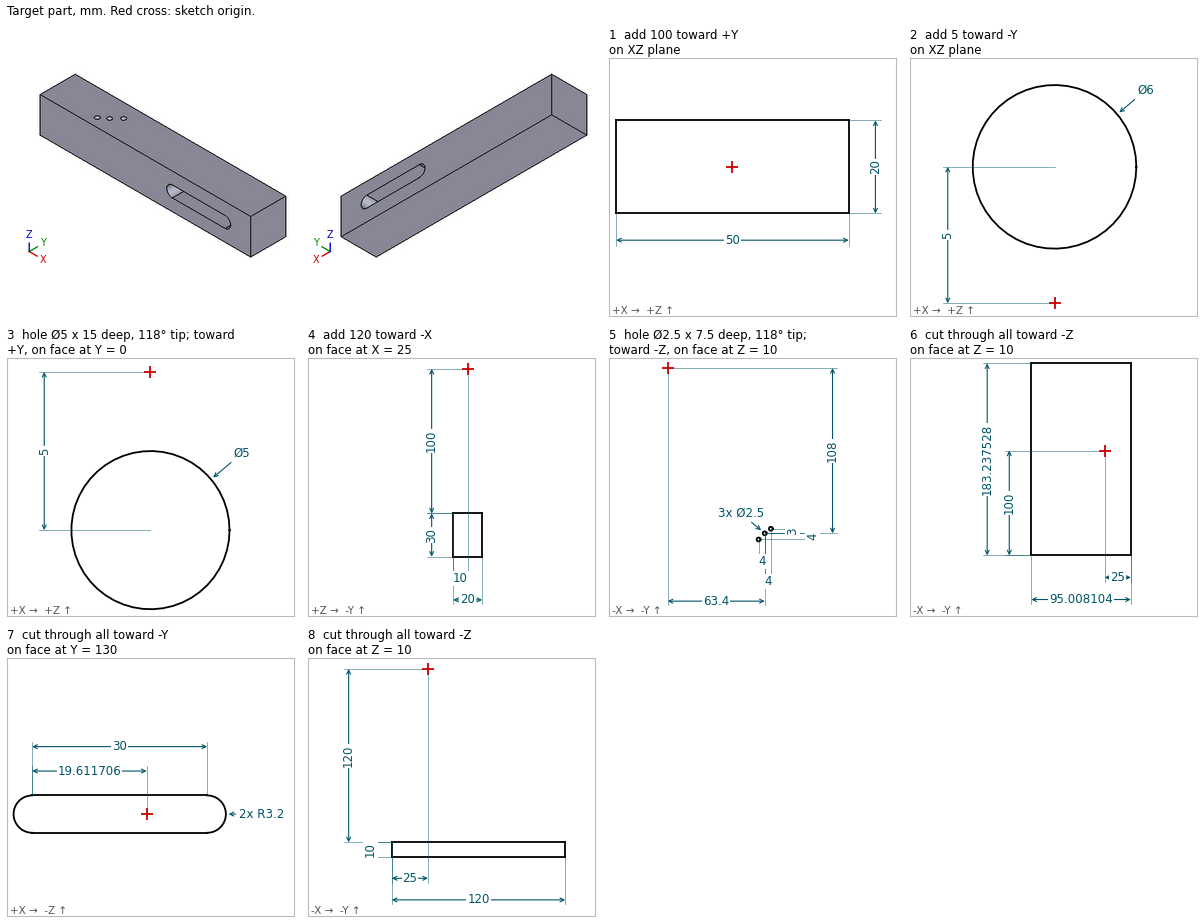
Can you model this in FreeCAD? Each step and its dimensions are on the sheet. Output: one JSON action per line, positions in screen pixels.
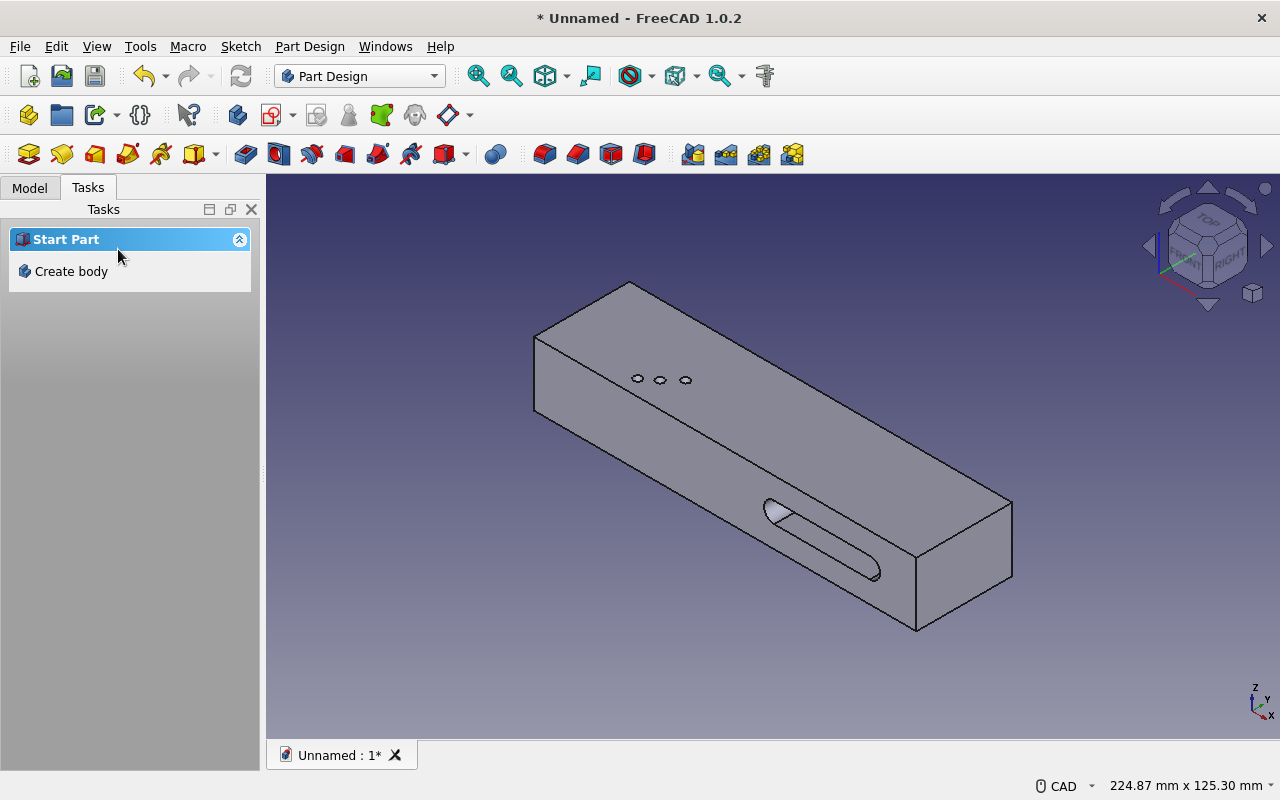
{"action": "left_click", "coordinate": [882, 482]}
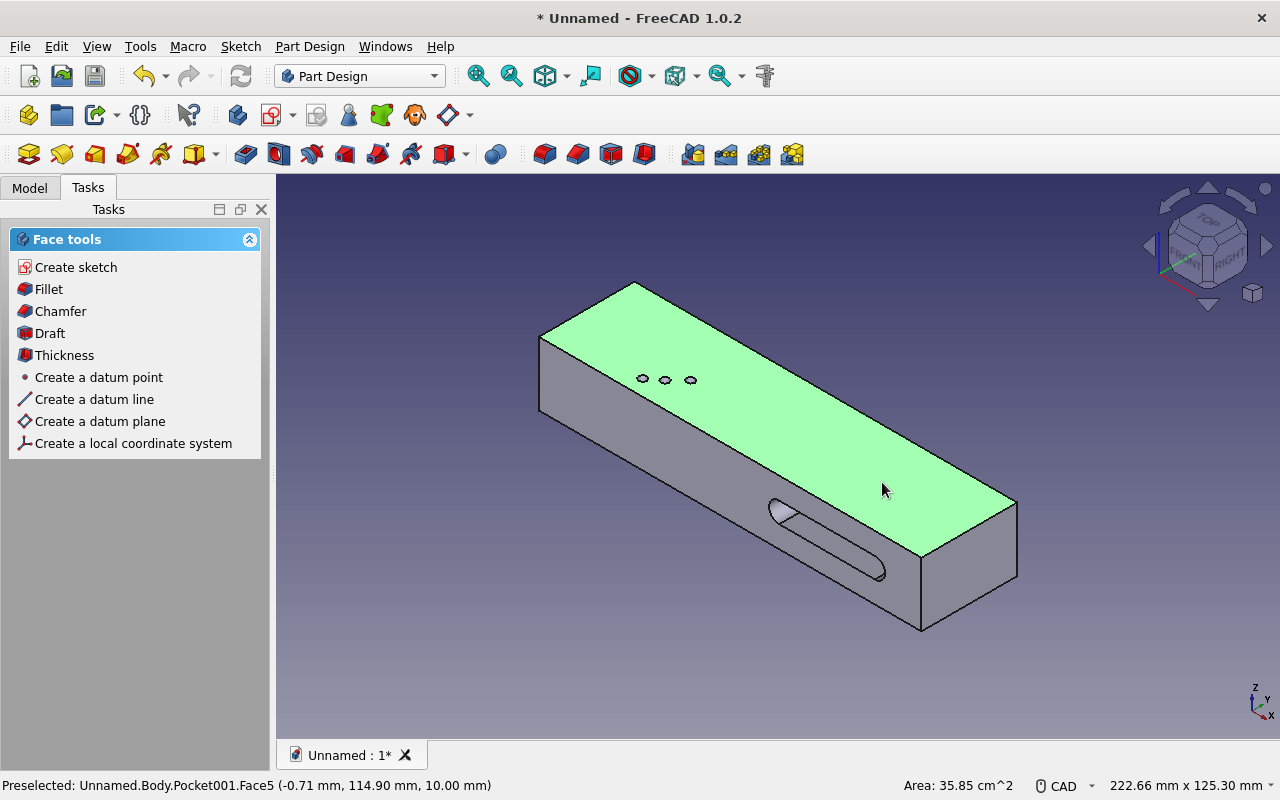
{"action": "left_click", "coordinate": [270, 116]}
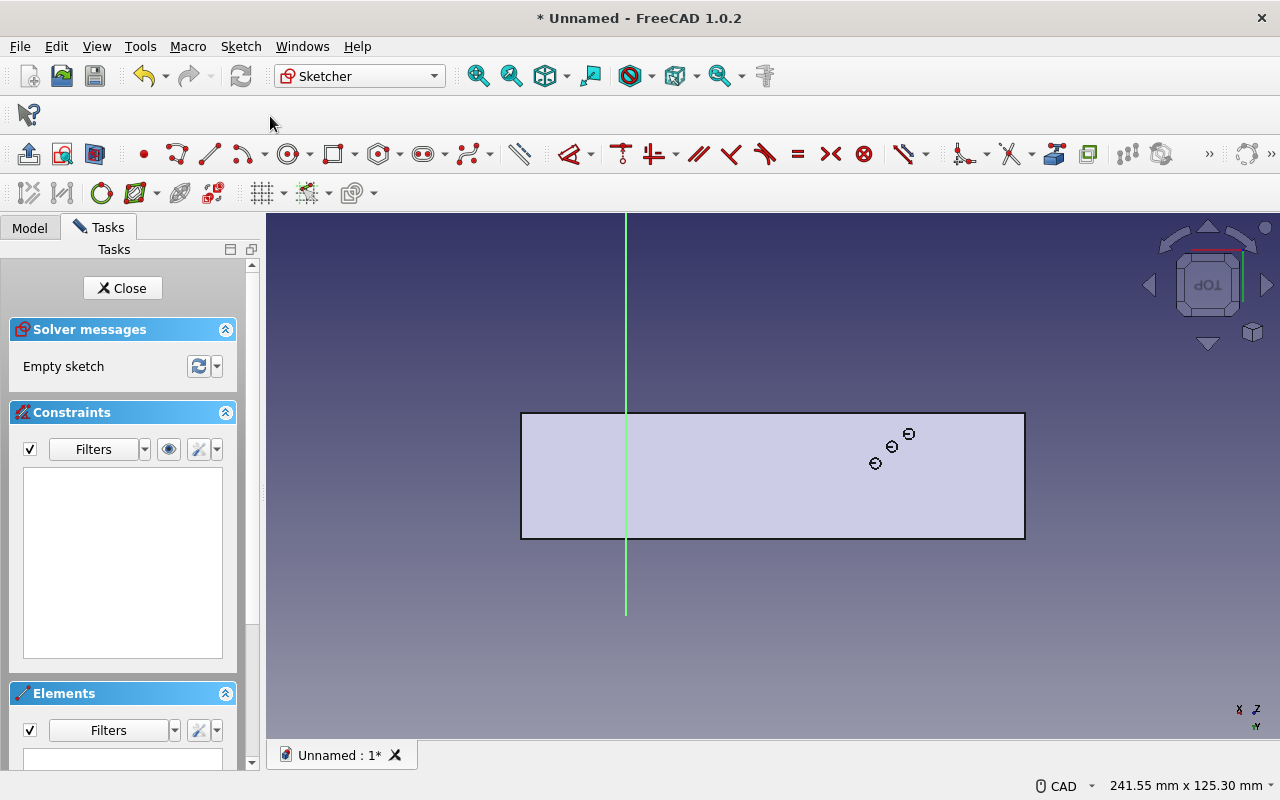
{"action": "scroll", "coordinate": [621, 711], "scroll_direction": "down", "scroll_amount": 3}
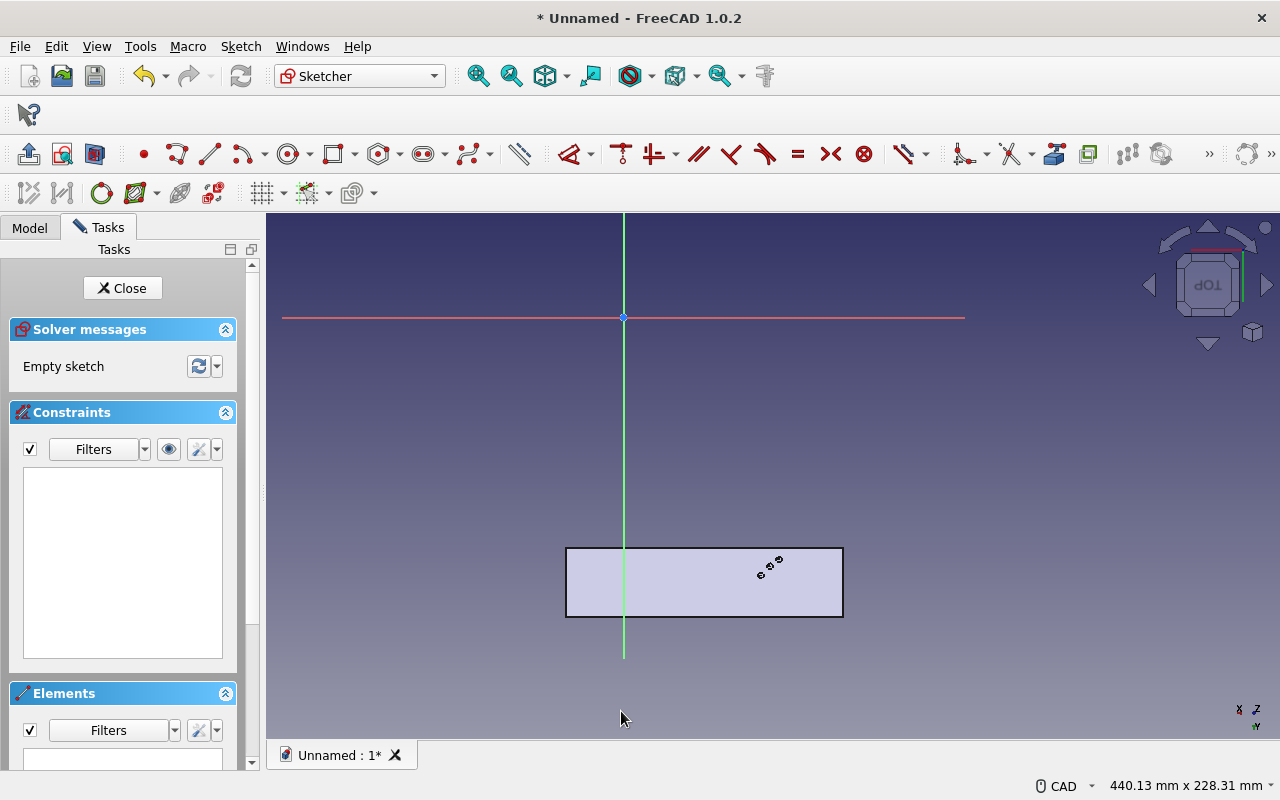
{"action": "left_click", "coordinate": [332, 154]}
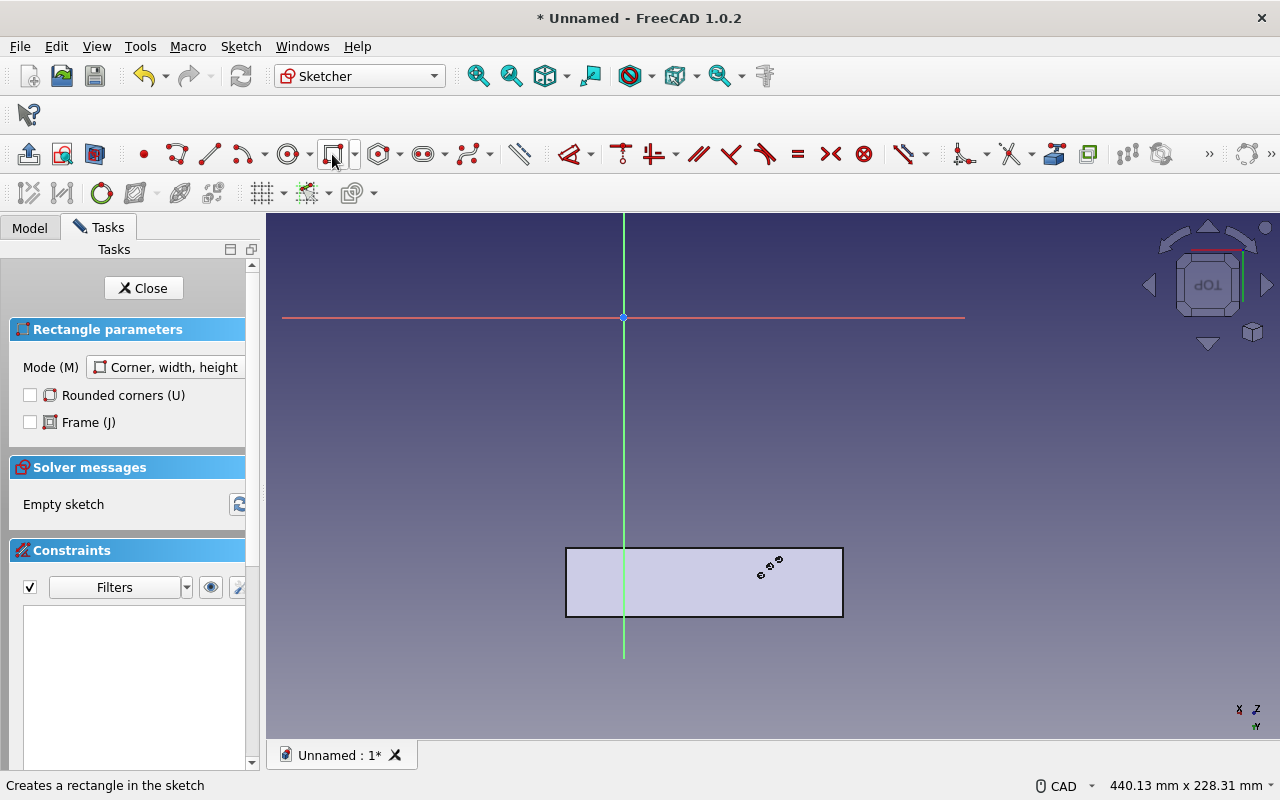
{"action": "left_click", "coordinate": [566, 594]}
{"action": "left_click", "coordinate": [843, 617]}
{"action": "key", "text": "Escape"}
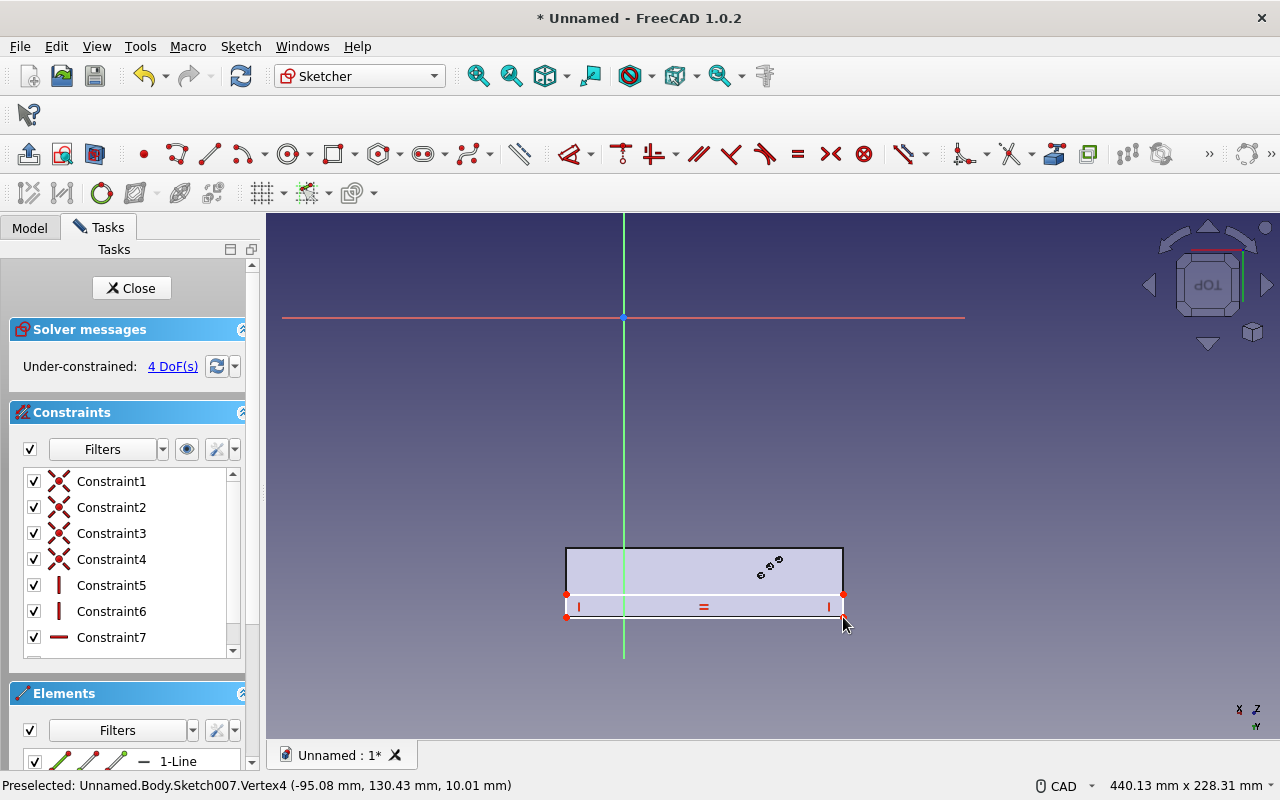
{"action": "left_click", "coordinate": [568, 154]}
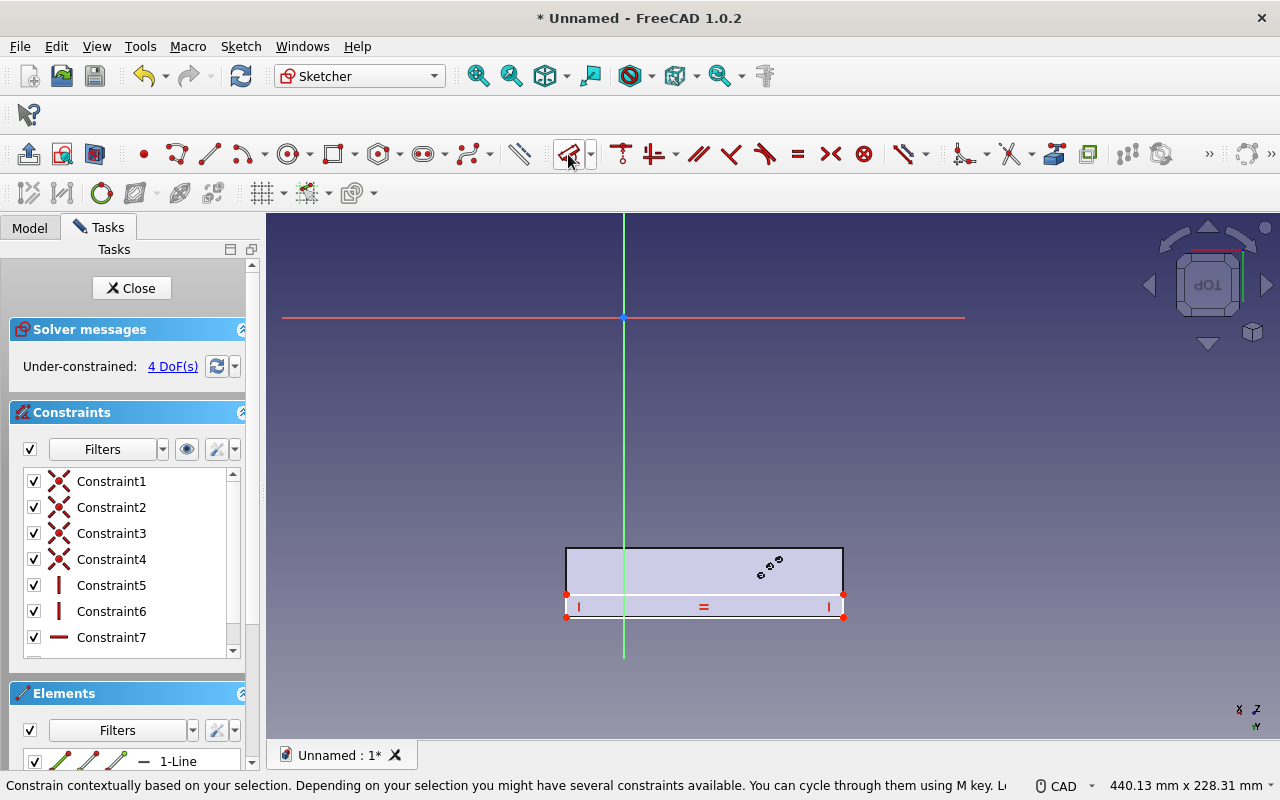
{"action": "scroll", "coordinate": [566, 604], "scroll_direction": "up", "scroll_amount": 3}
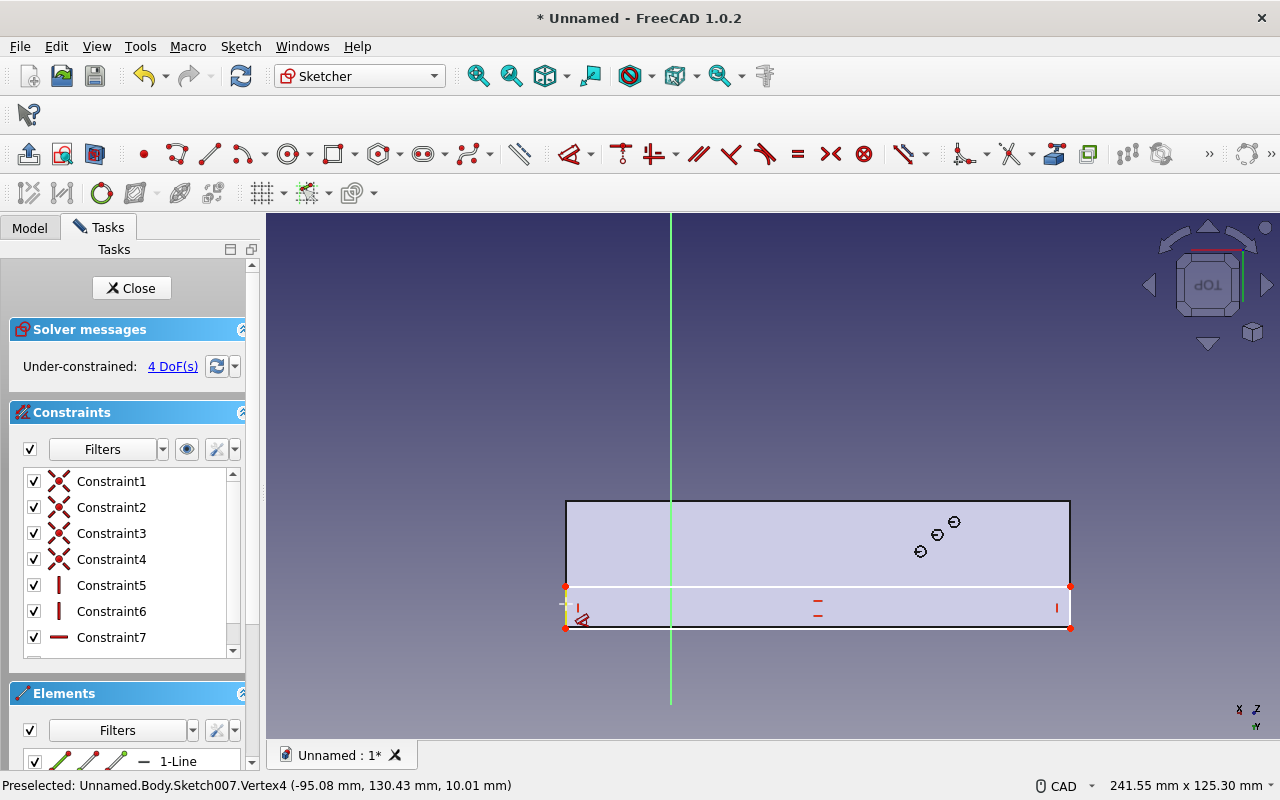
{"action": "left_click", "coordinate": [566, 604]}
{"action": "left_click", "coordinate": [532, 608]}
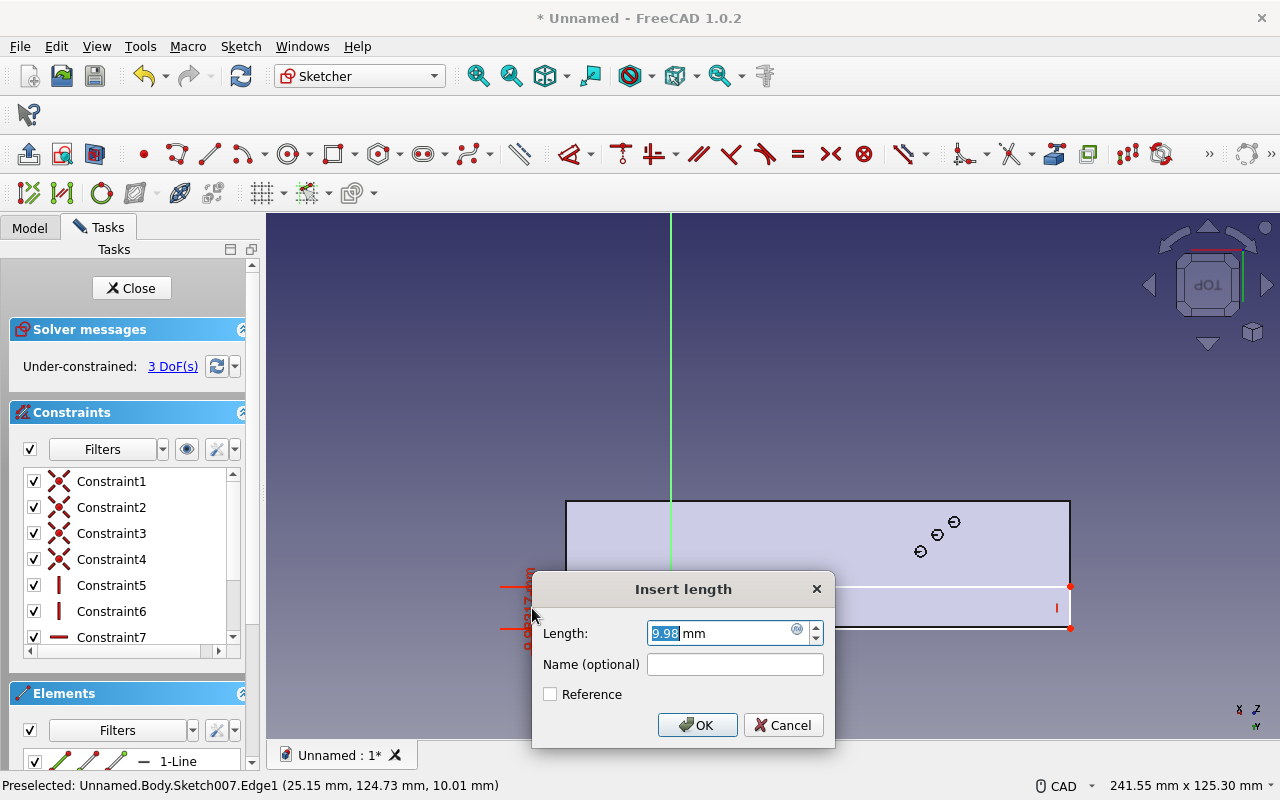
{"action": "type", "text": "10"}
{"action": "key", "text": "Return"}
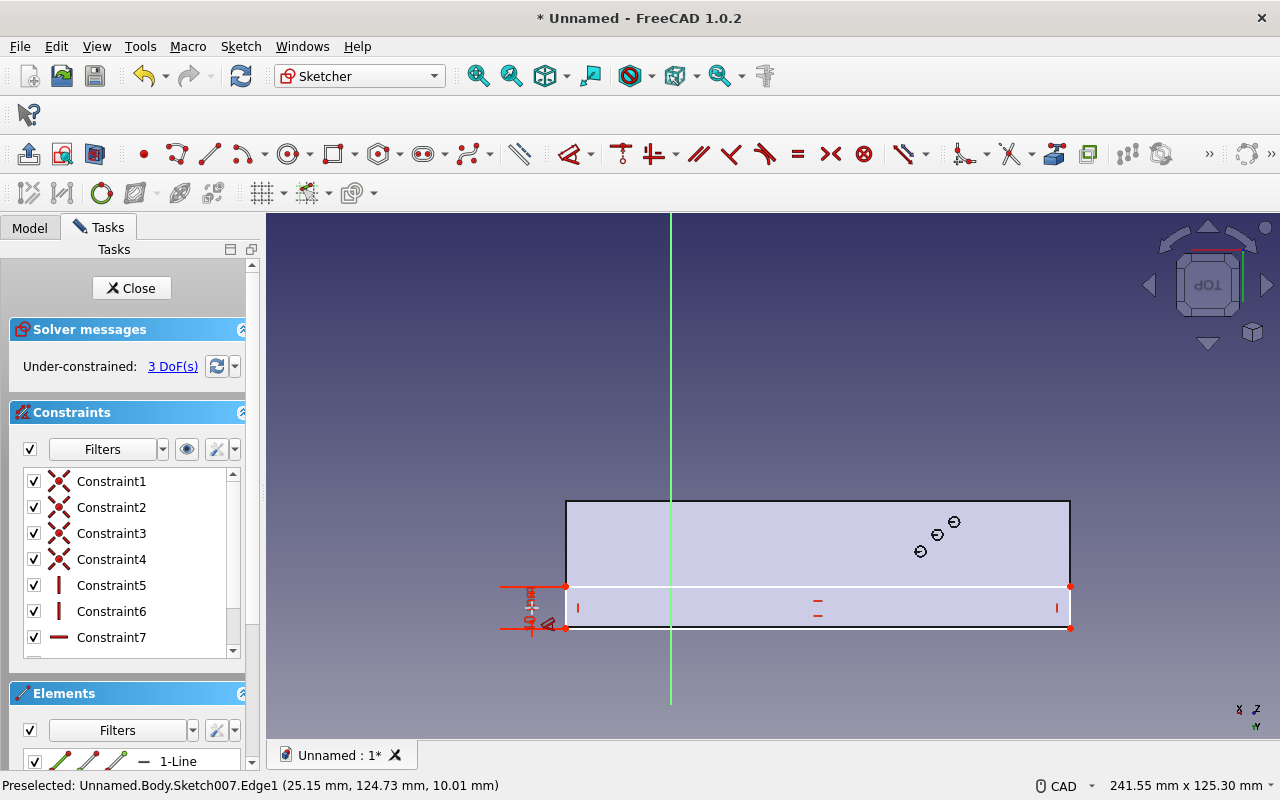
{"action": "left_click", "coordinate": [717, 629]}
{"action": "left_click", "coordinate": [818, 663]}